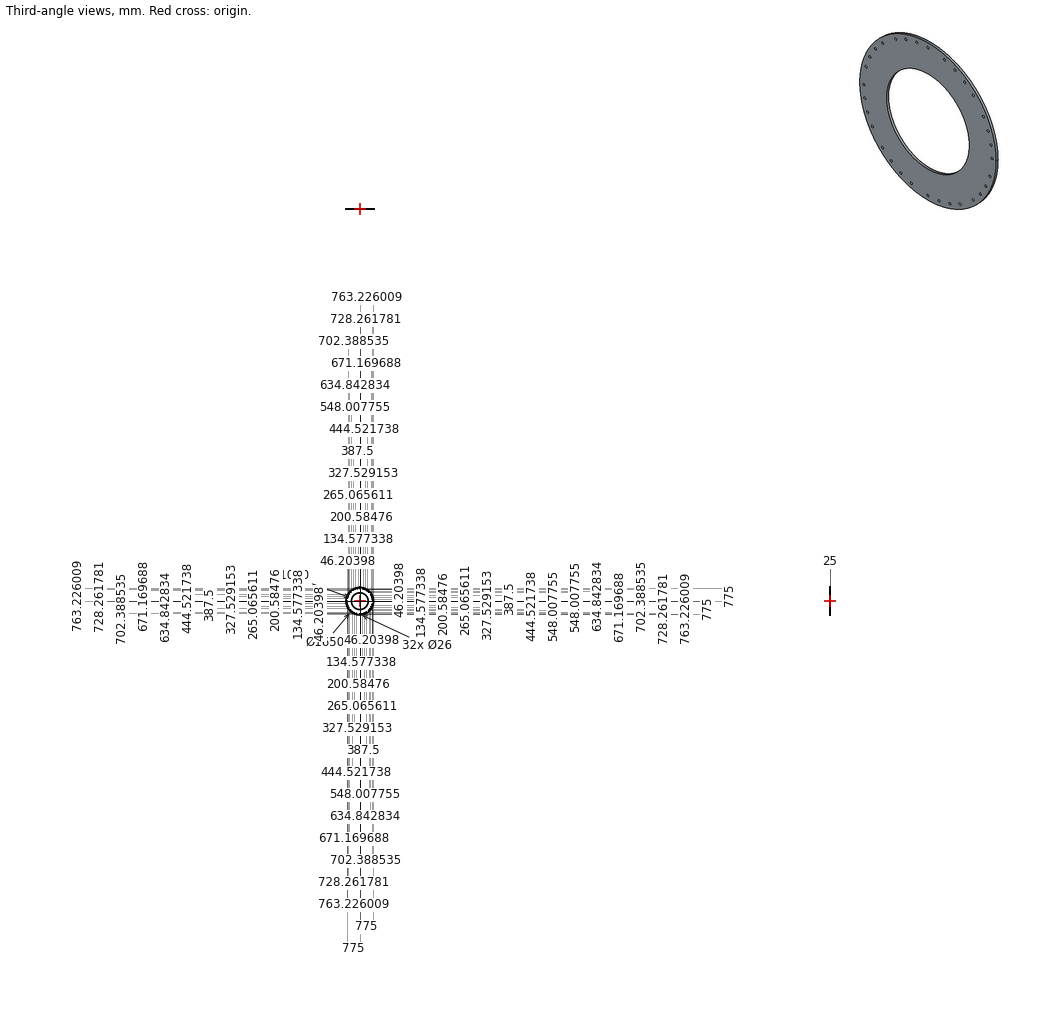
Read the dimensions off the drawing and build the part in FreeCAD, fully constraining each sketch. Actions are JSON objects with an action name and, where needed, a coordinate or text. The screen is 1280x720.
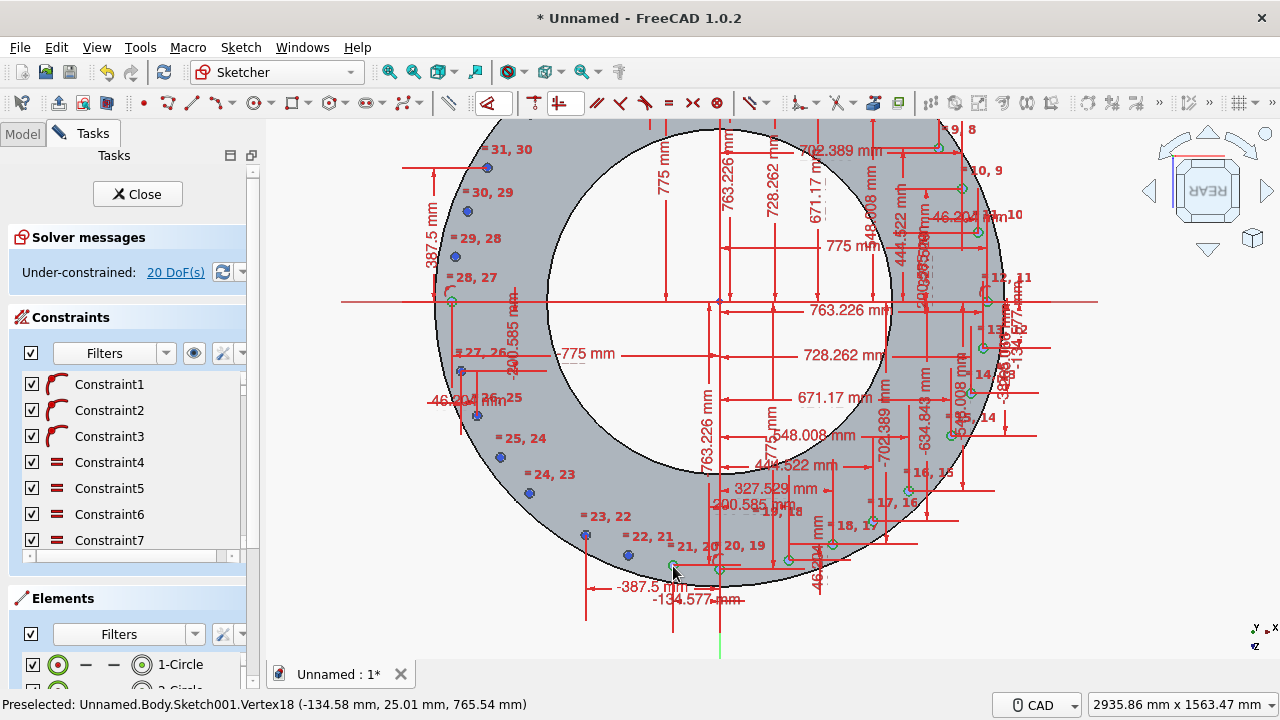
{"action": "left_click", "coordinate": [628, 555]}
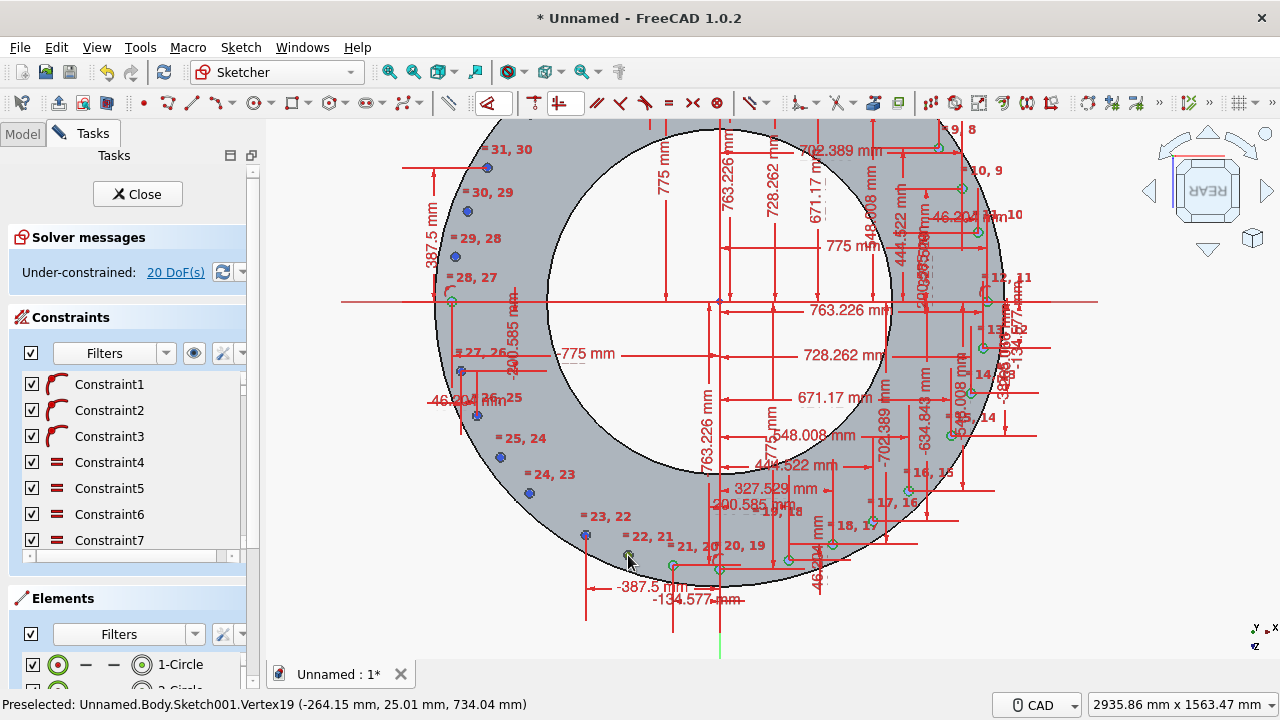
{"action": "left_click", "coordinate": [506, 104]}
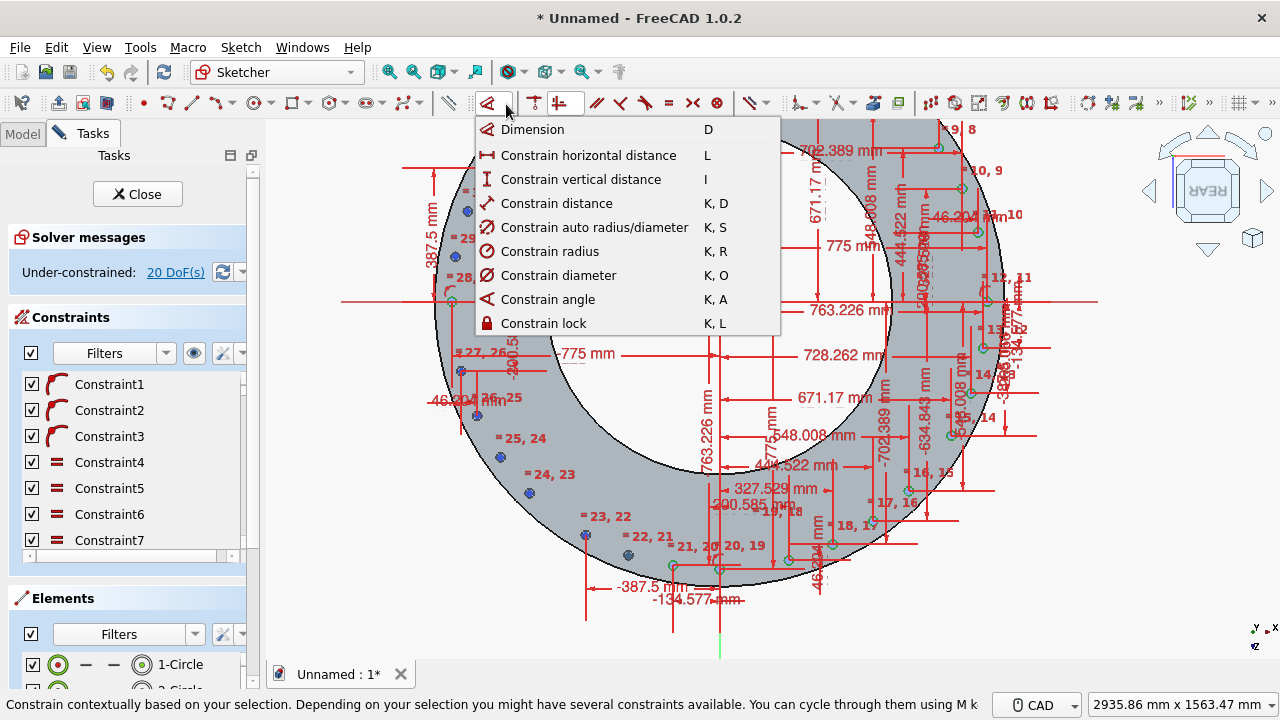
{"action": "left_click", "coordinate": [628, 155]}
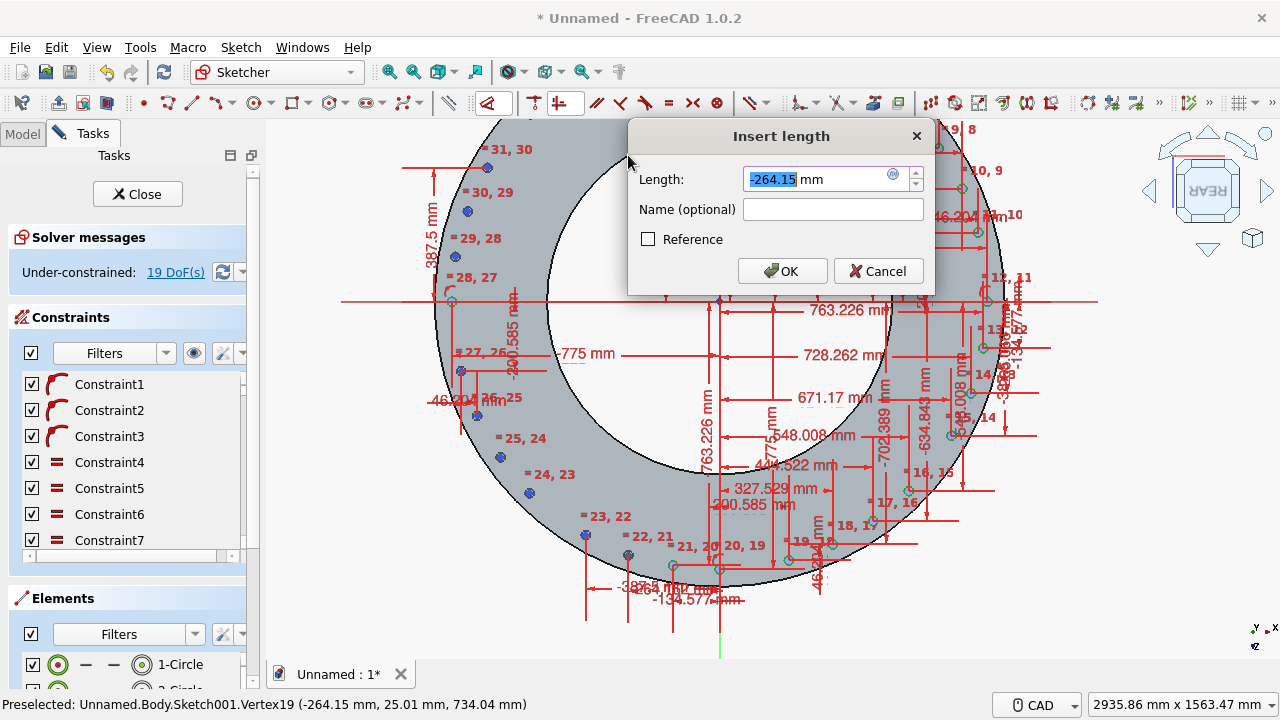
{"action": "type", "text": "-265.065611"}
{"action": "key", "text": "Return"}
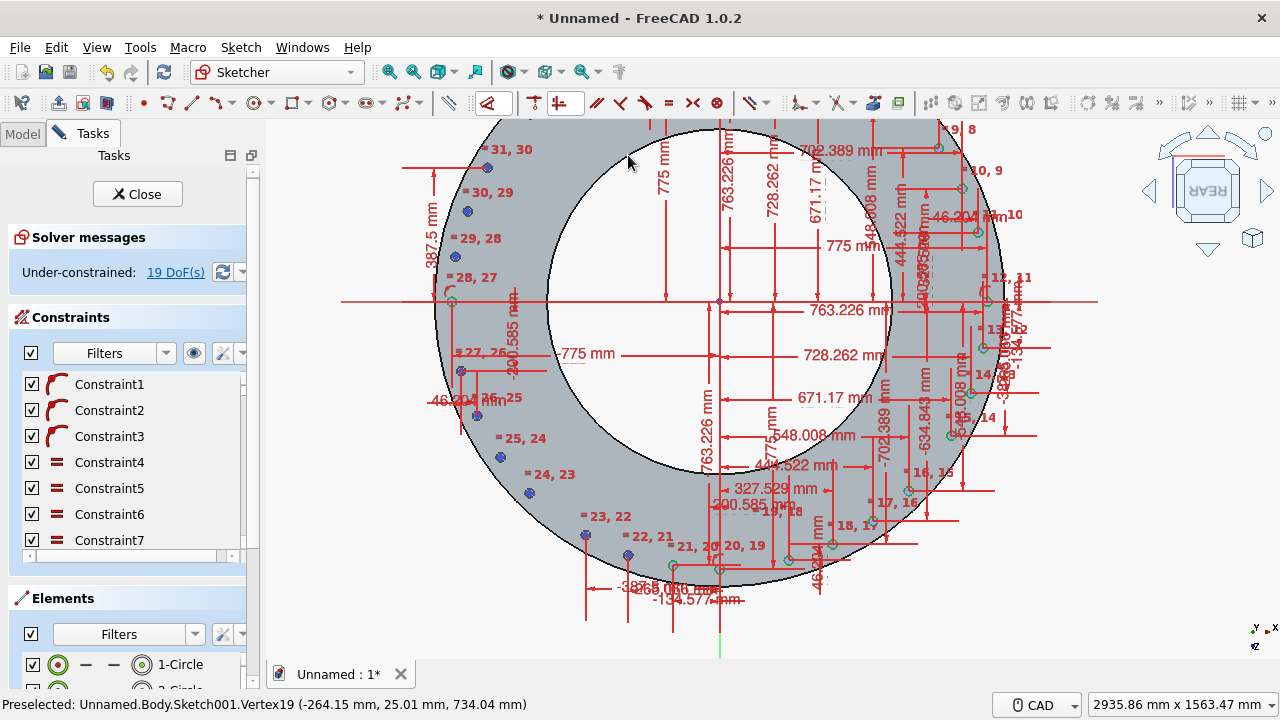
{"action": "left_click", "coordinate": [628, 555]}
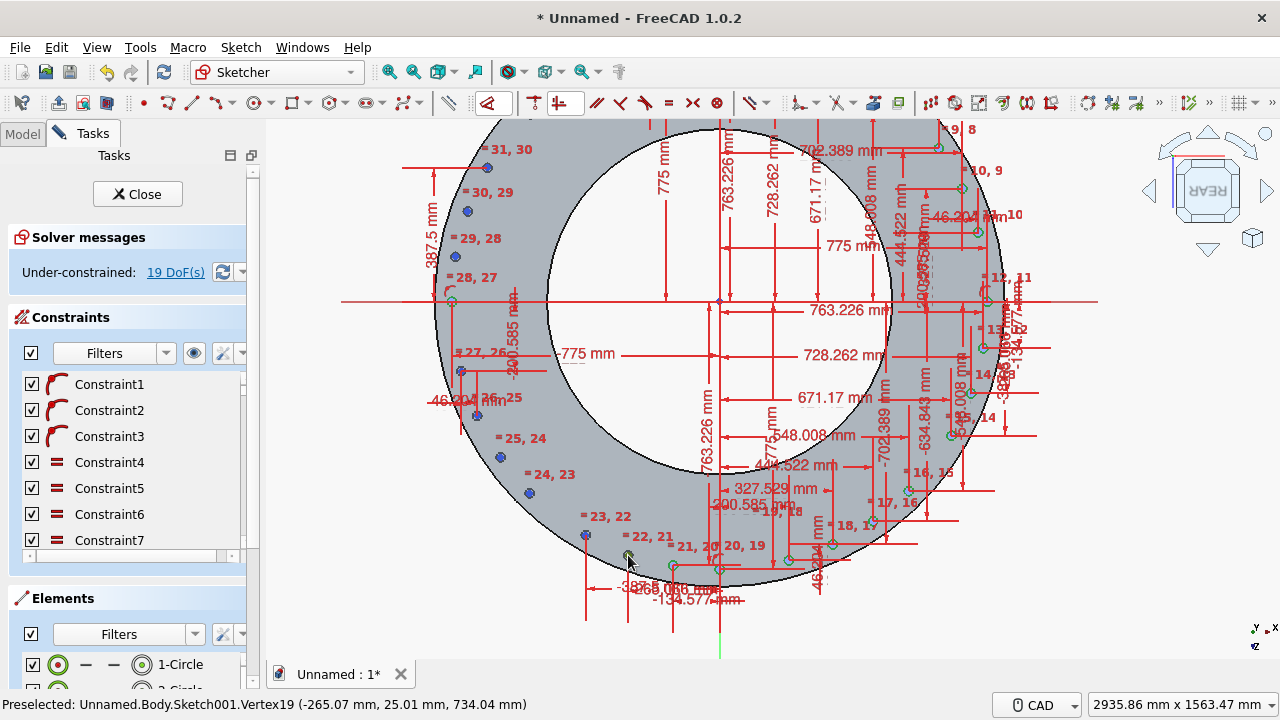
{"action": "left_click", "coordinate": [506, 104]}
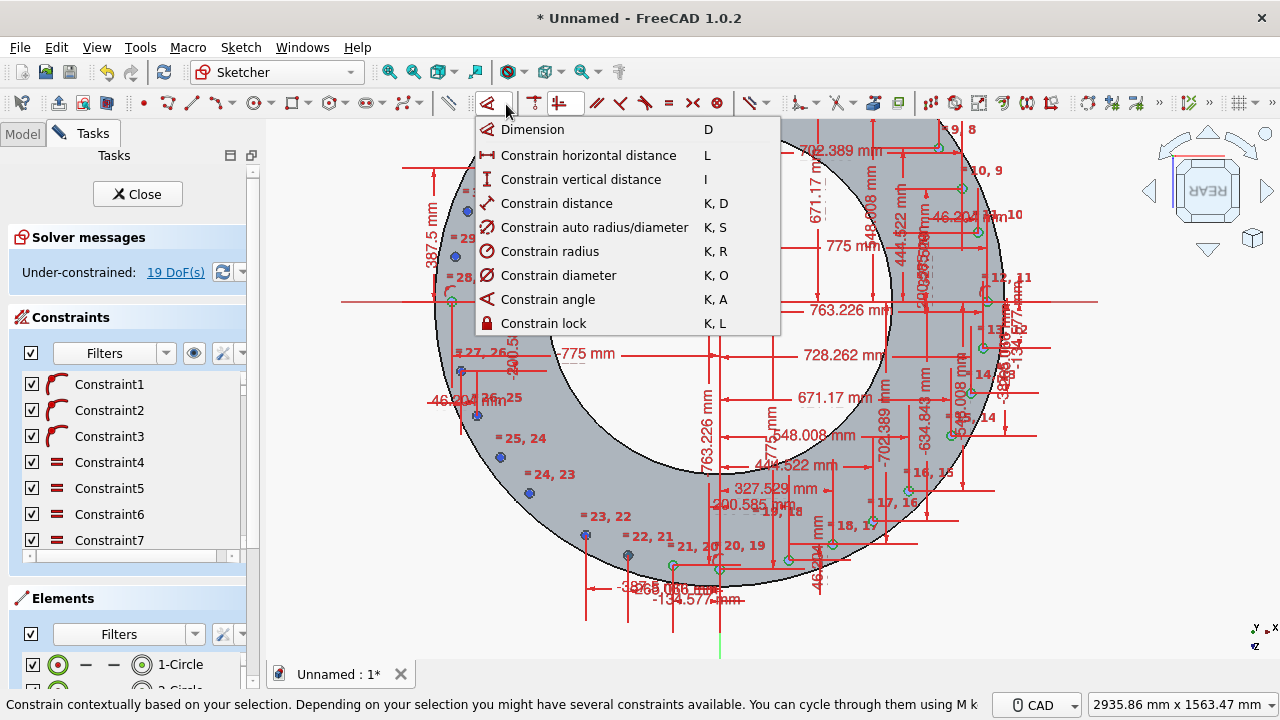
{"action": "left_click", "coordinate": [628, 179]}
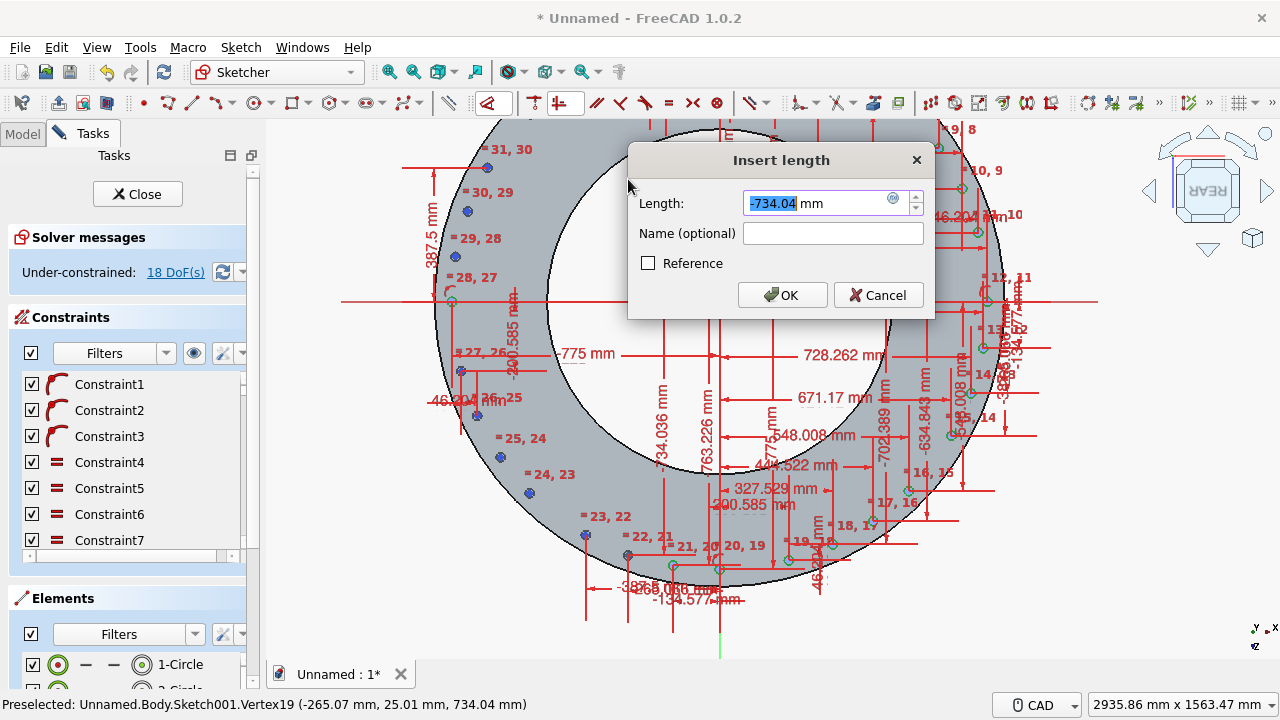
{"action": "type", "text": "-728.261781"}
{"action": "key", "text": "Return"}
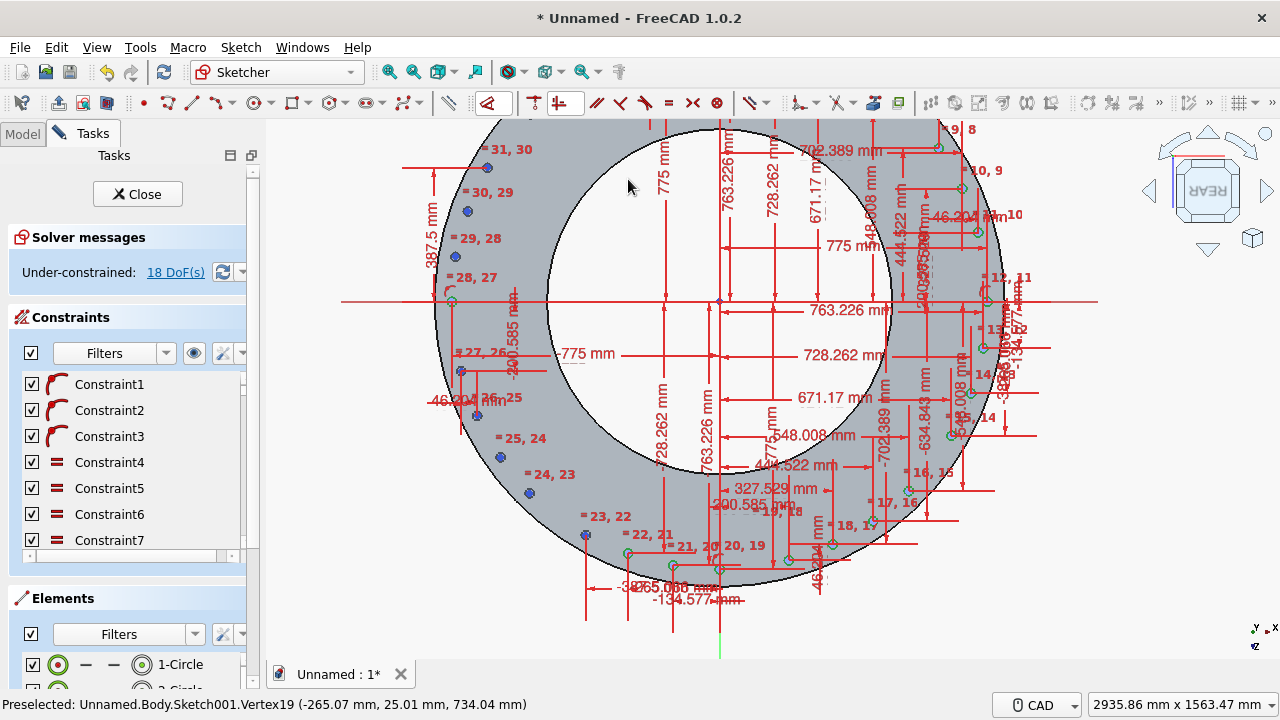
{"action": "left_click", "coordinate": [586, 535]}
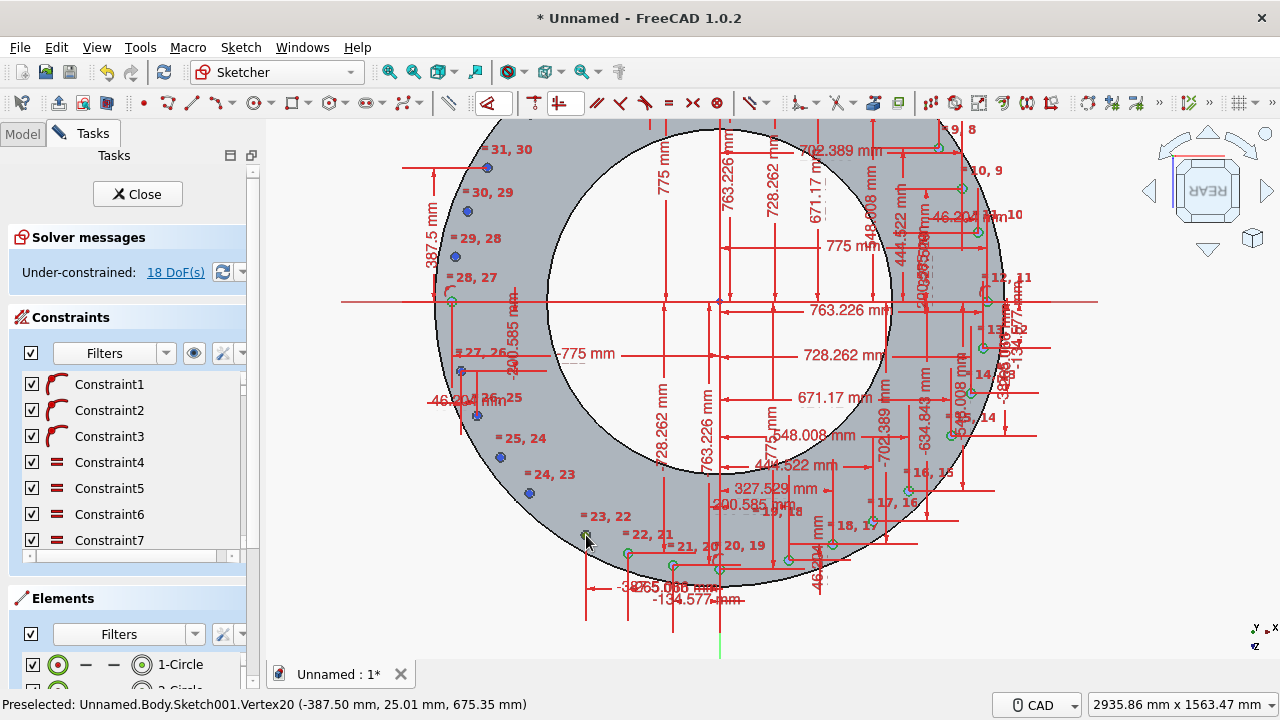
{"action": "left_click", "coordinate": [506, 104]}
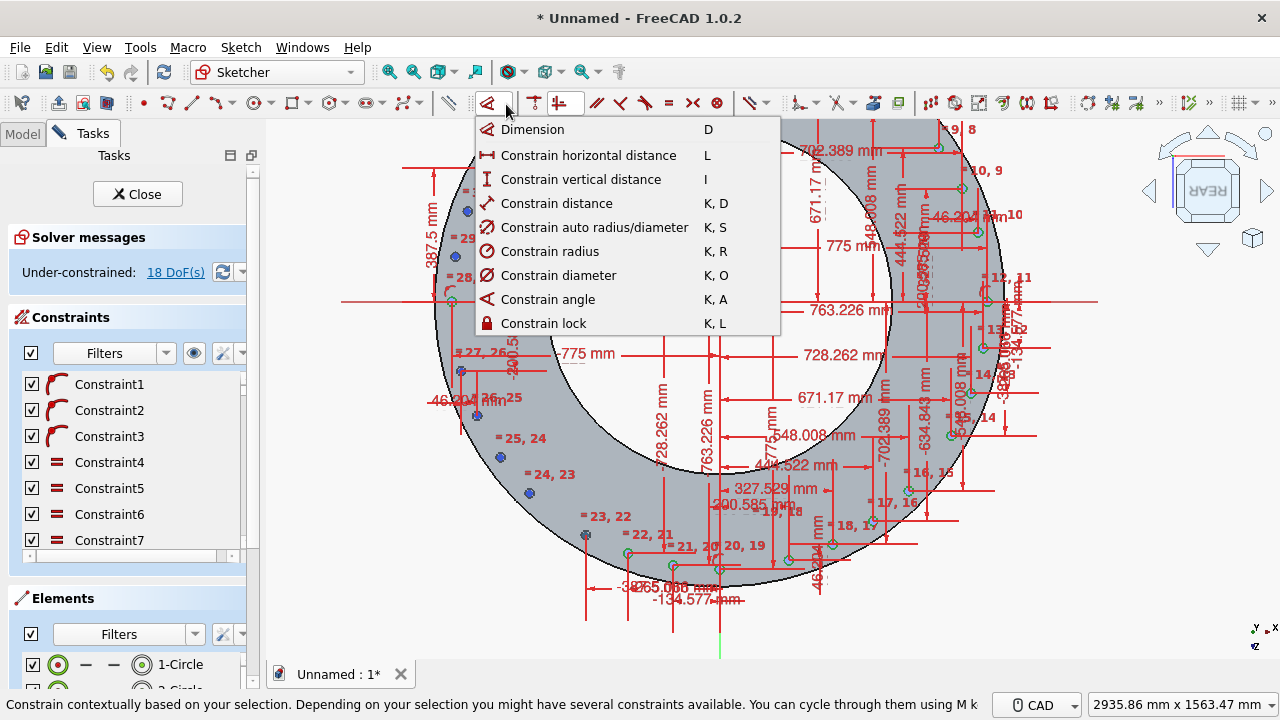
{"action": "left_click", "coordinate": [628, 179]}